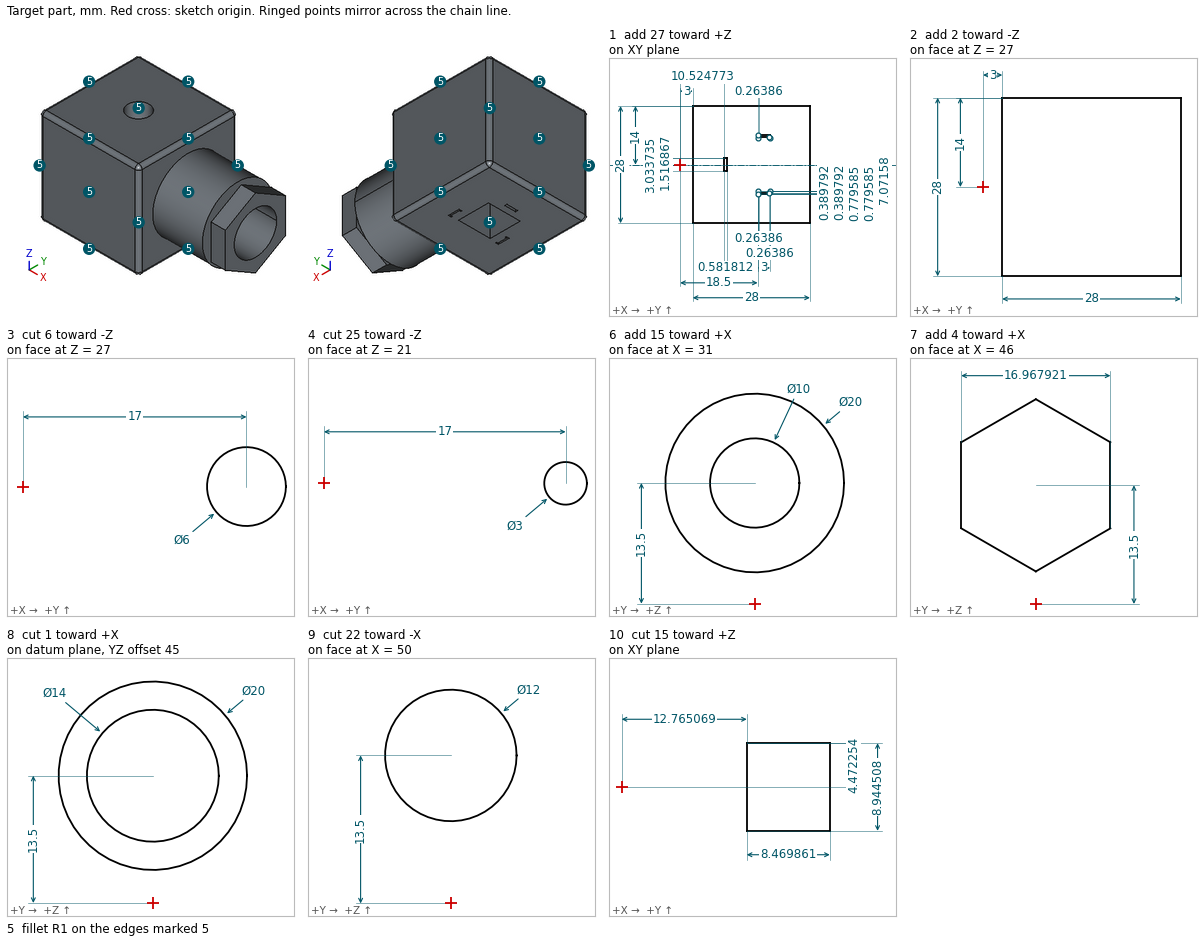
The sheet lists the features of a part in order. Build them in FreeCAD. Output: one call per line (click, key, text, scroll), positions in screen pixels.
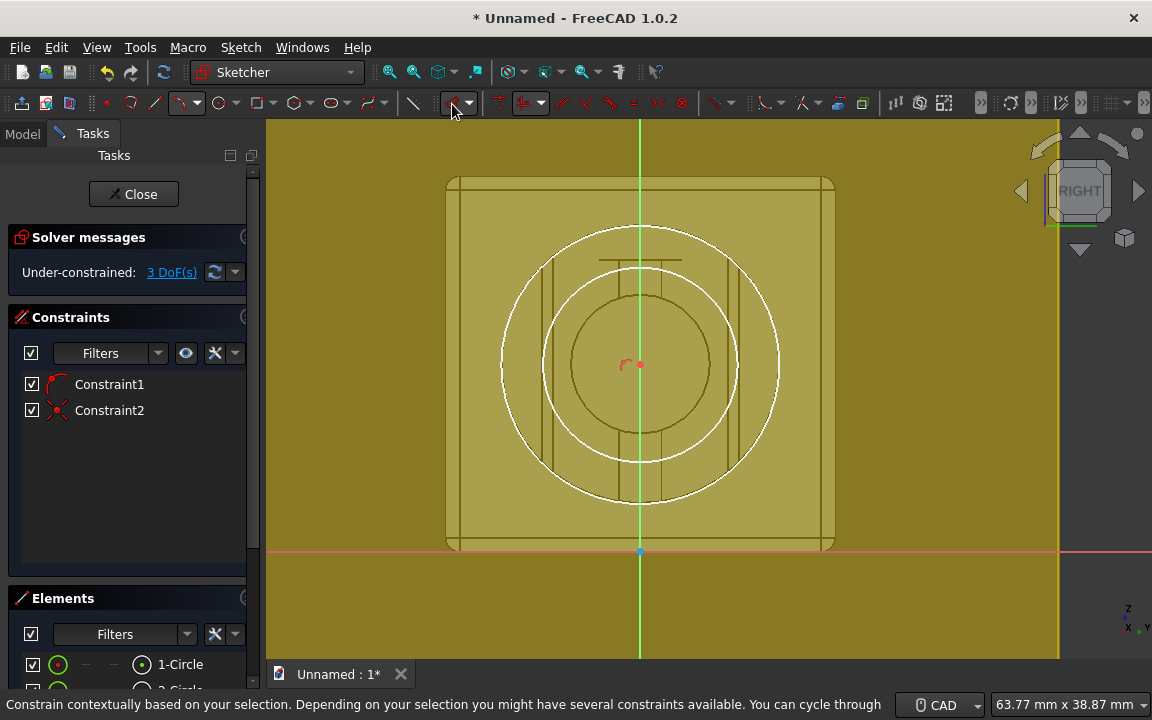
click(738, 266)
click(760, 243)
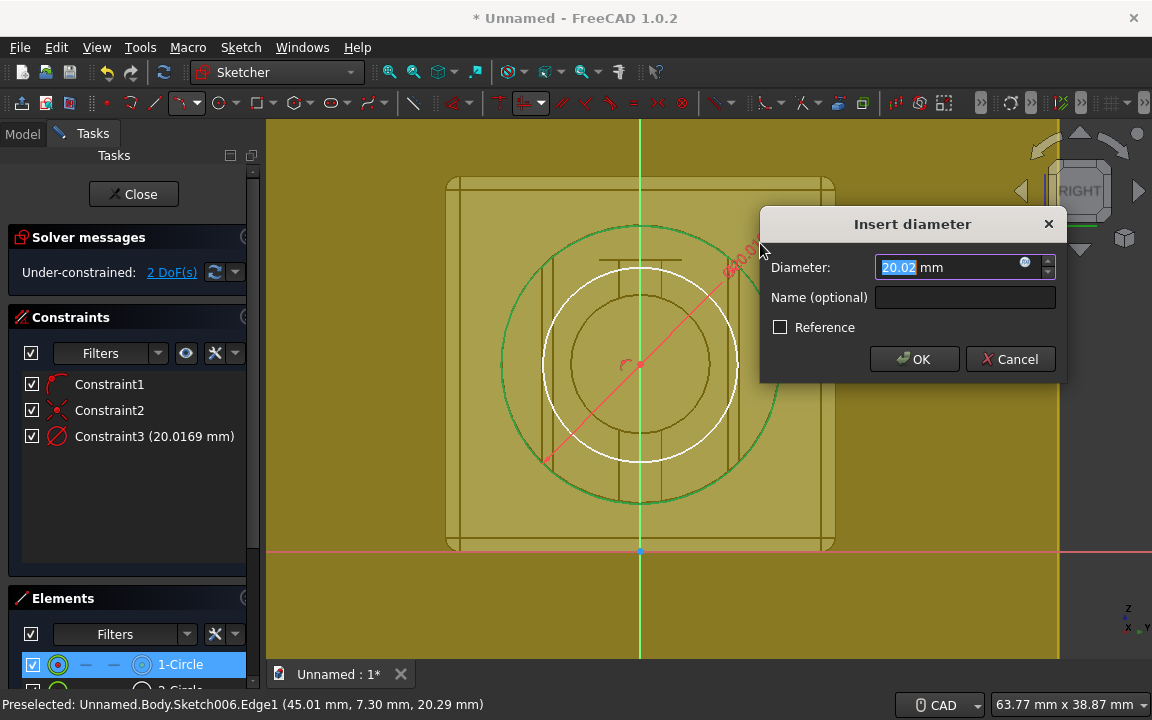
text(20)
key(Return)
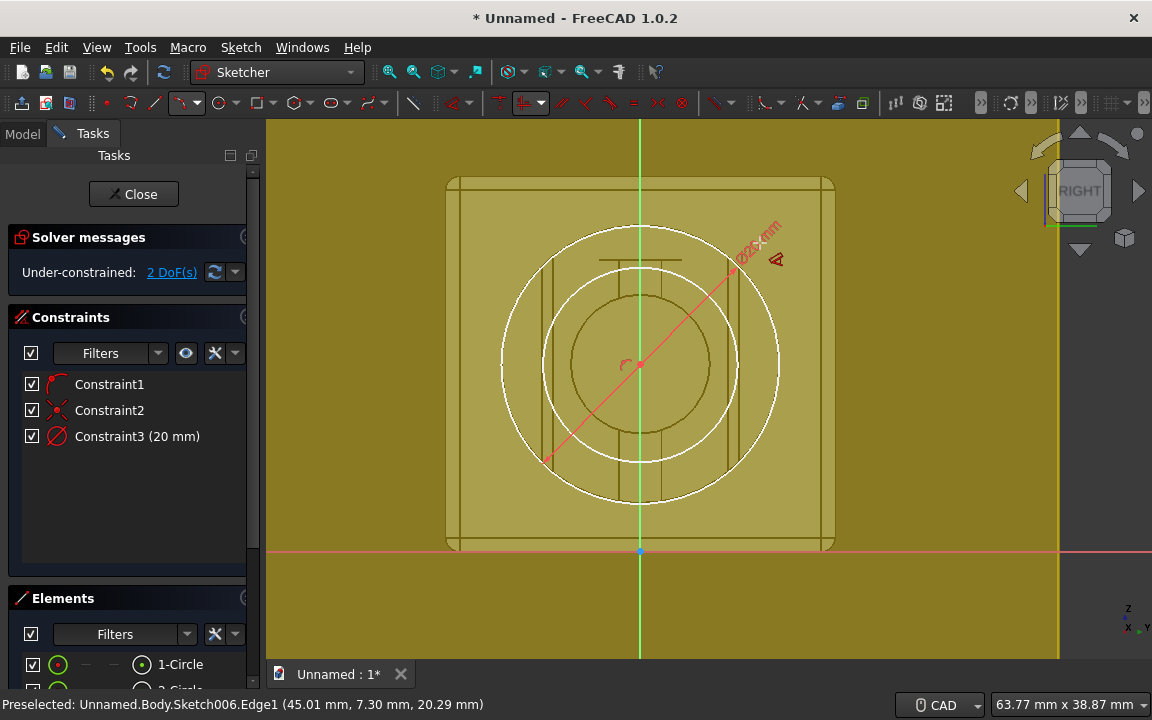
click(709, 296)
click(786, 322)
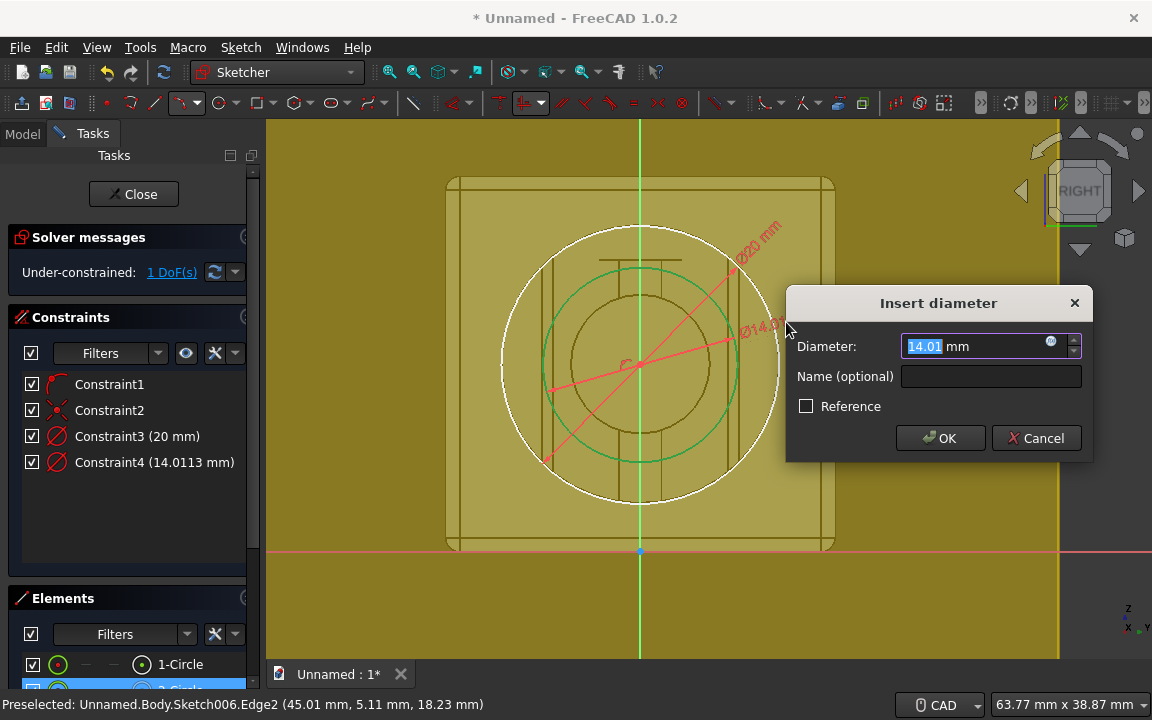
text(14)
key(Return)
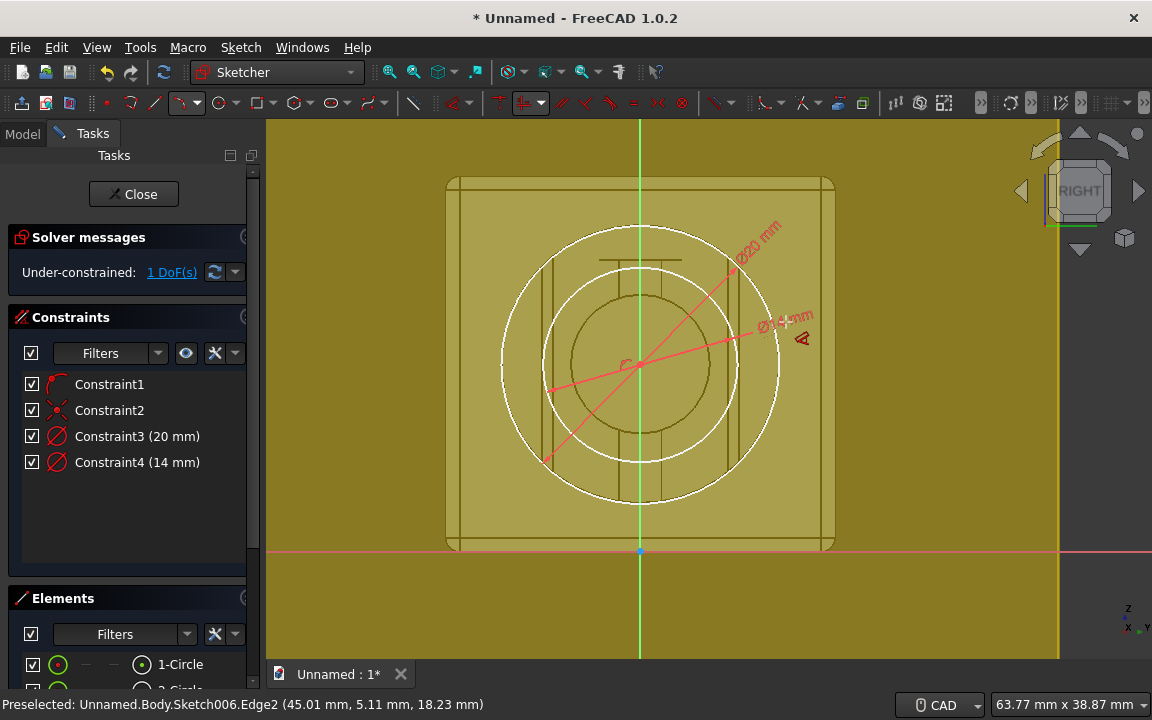
click(640, 365)
click(674, 415)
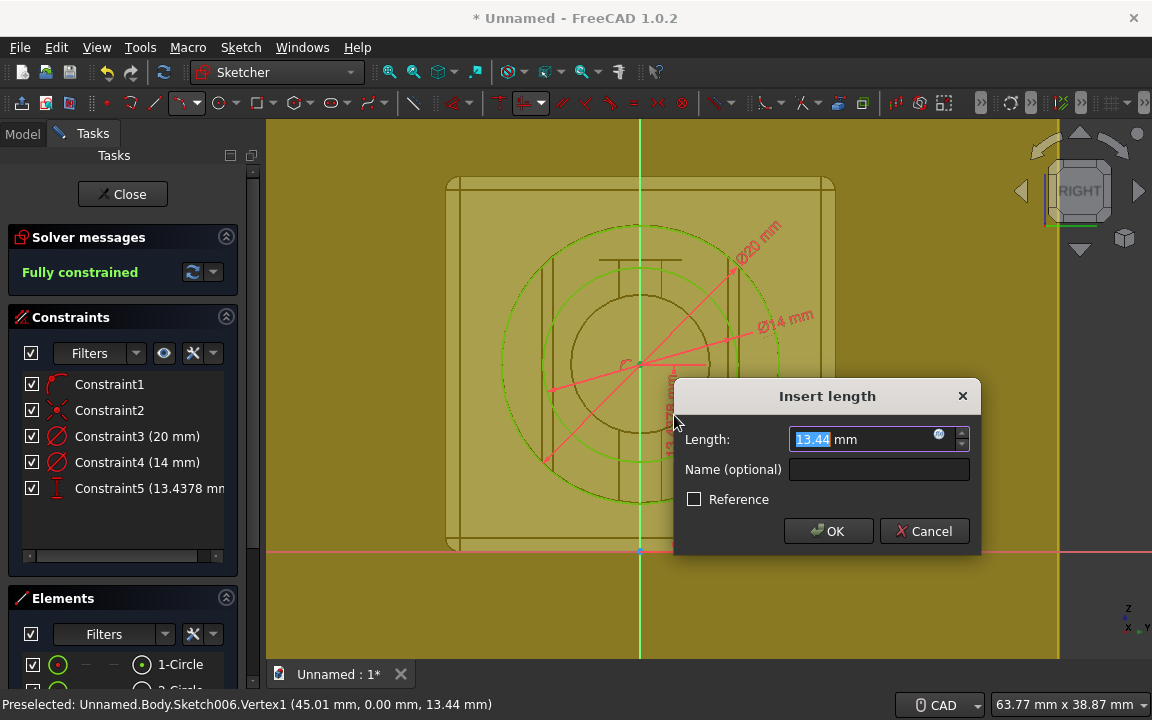
text(13.5)
key(Return)
key(Escape)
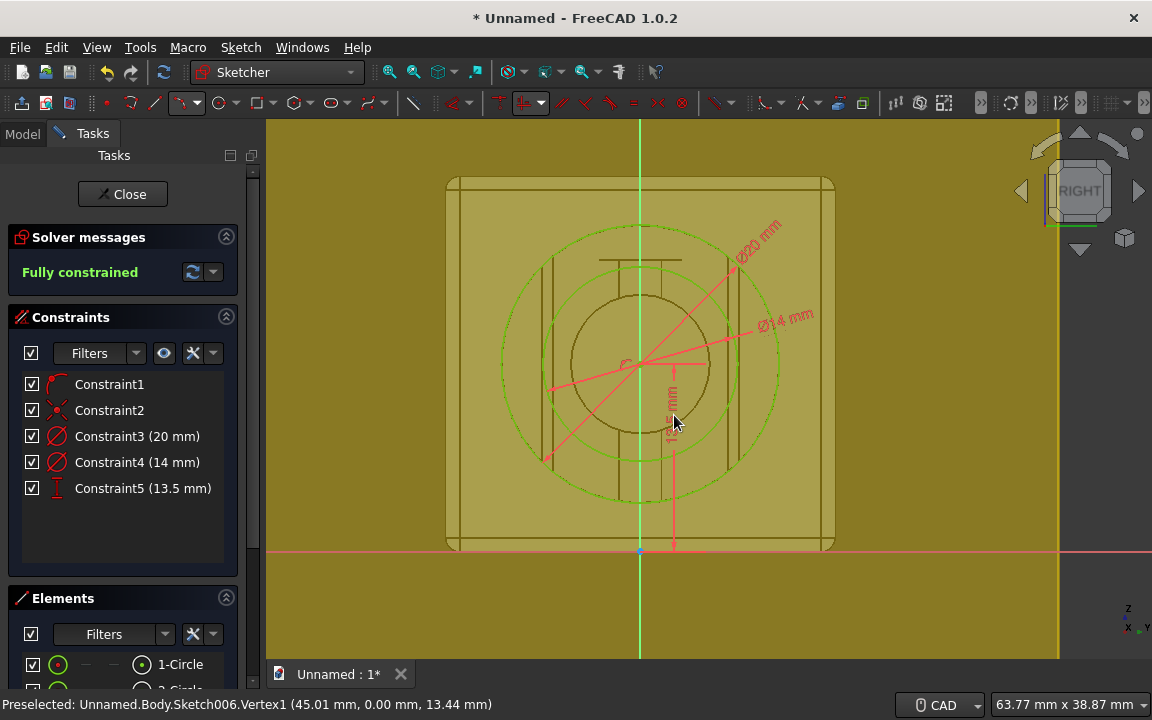
click(123, 194)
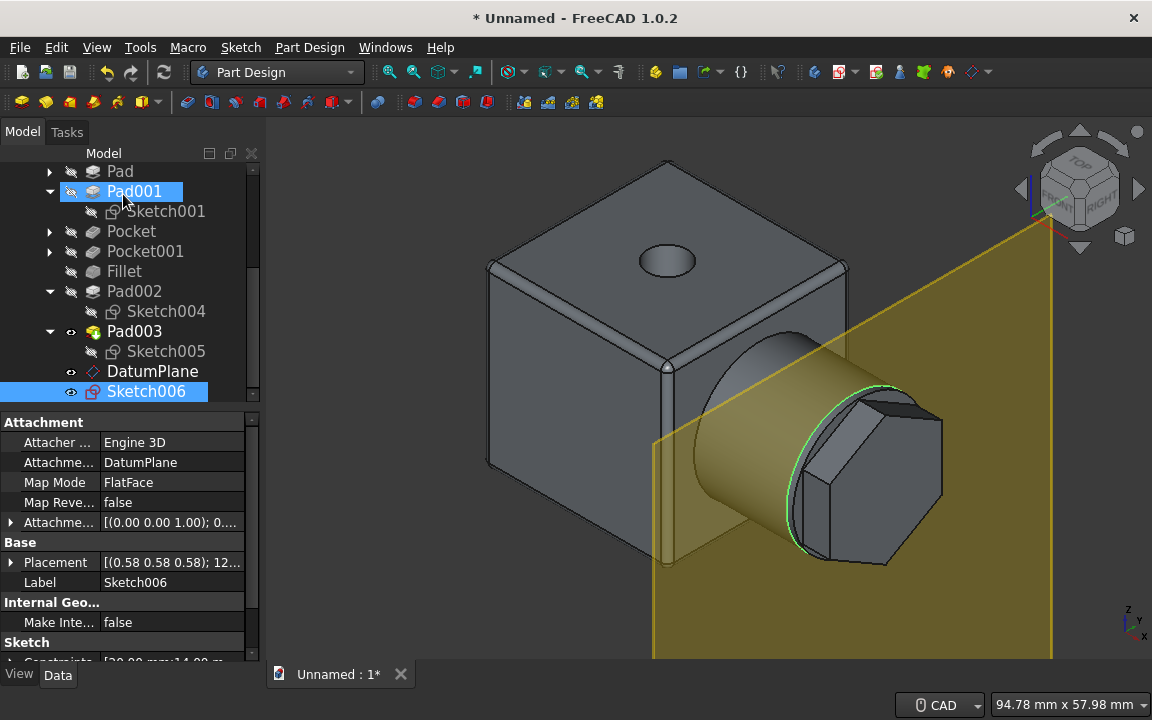
click(188, 102)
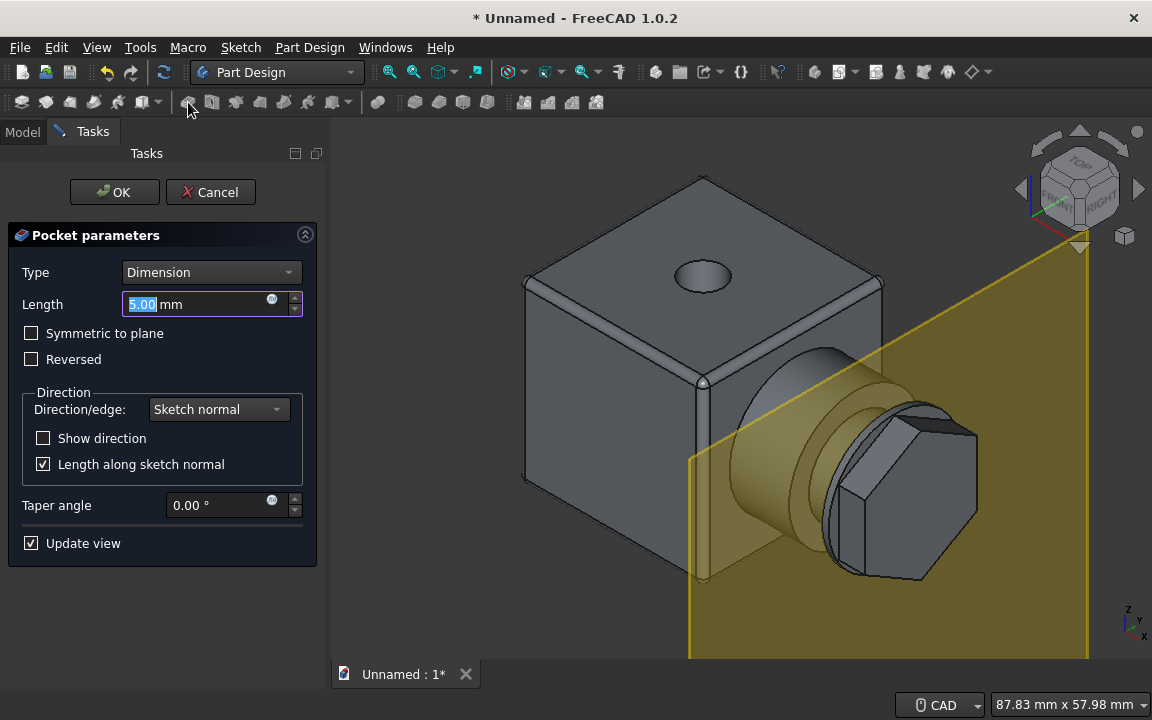
text(1)
key(Tab)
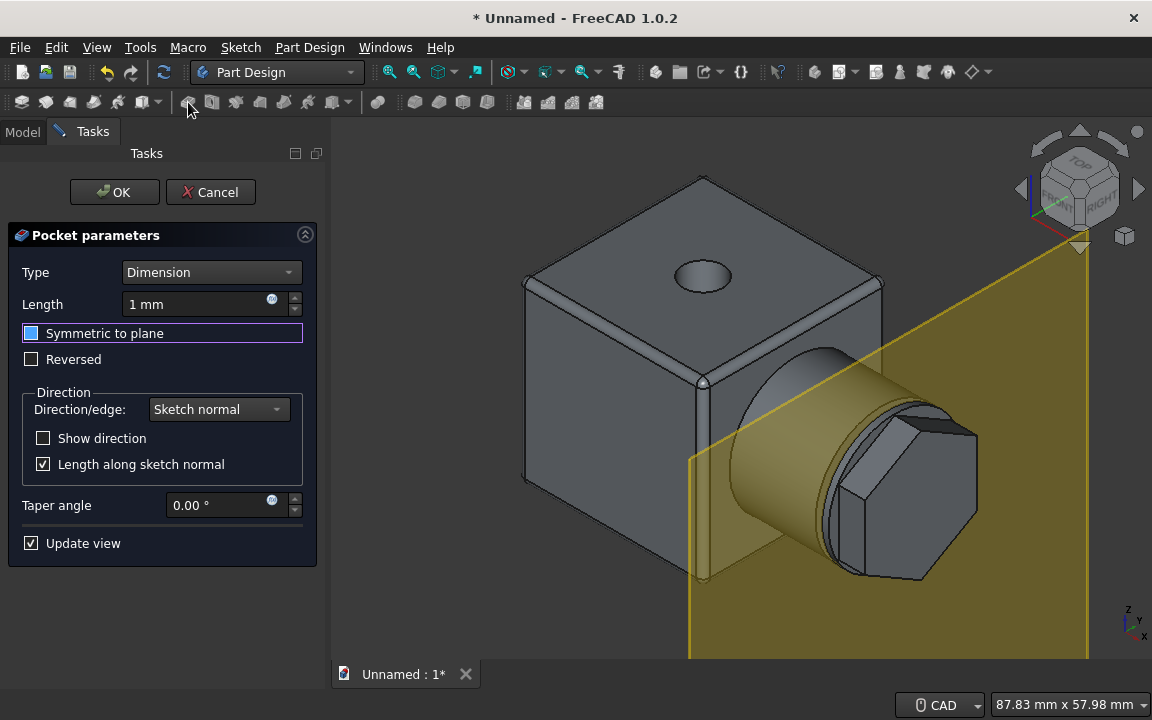
click(30, 359)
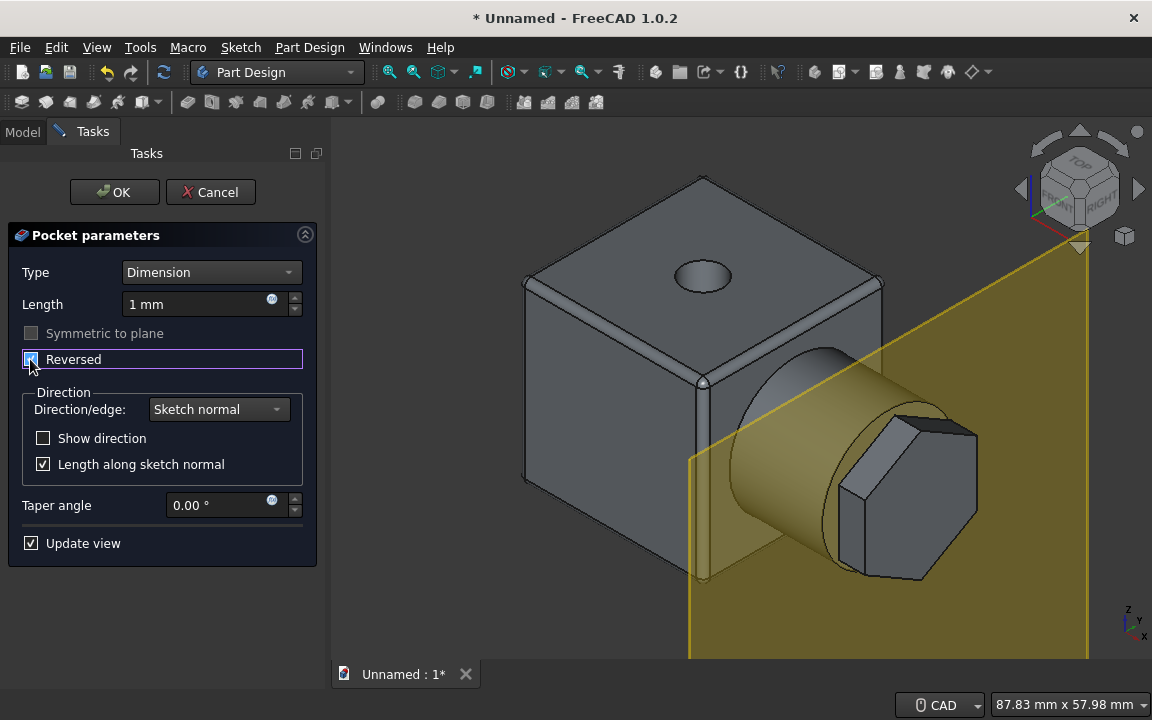
click(115, 192)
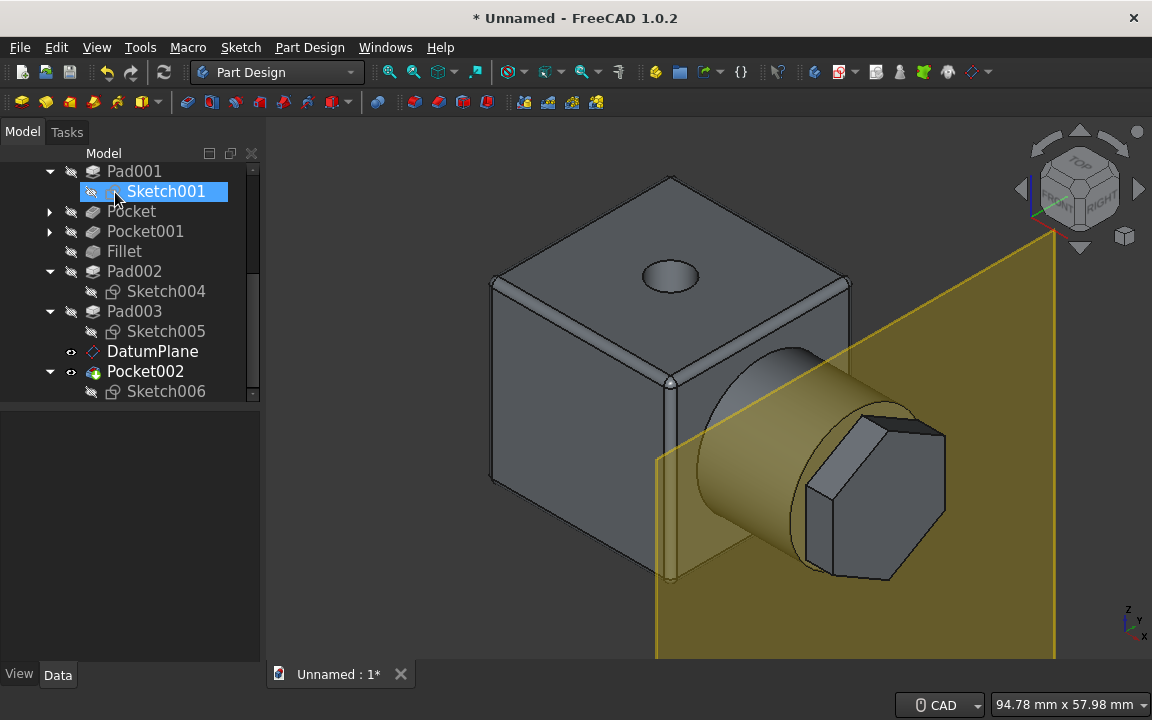
click(116, 352)
key(space)